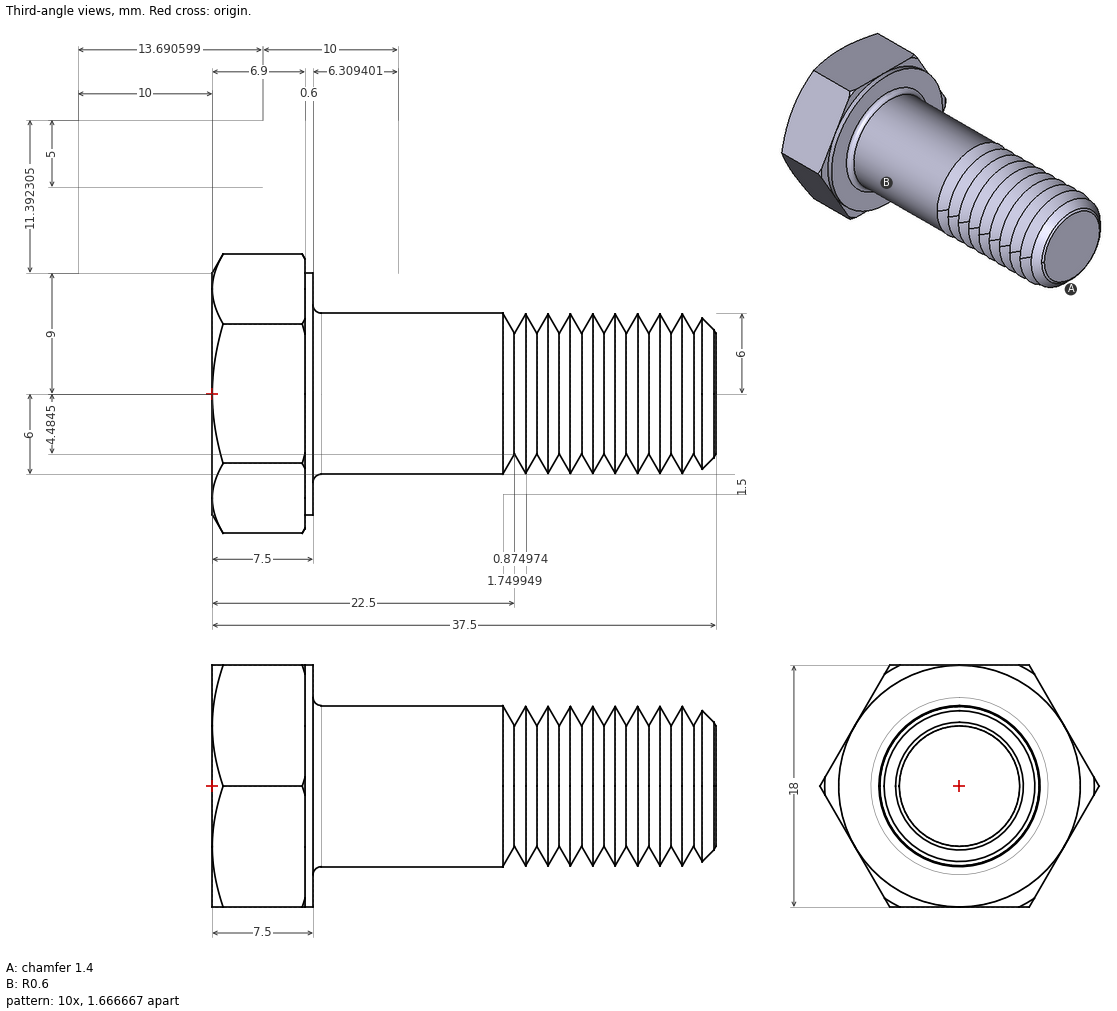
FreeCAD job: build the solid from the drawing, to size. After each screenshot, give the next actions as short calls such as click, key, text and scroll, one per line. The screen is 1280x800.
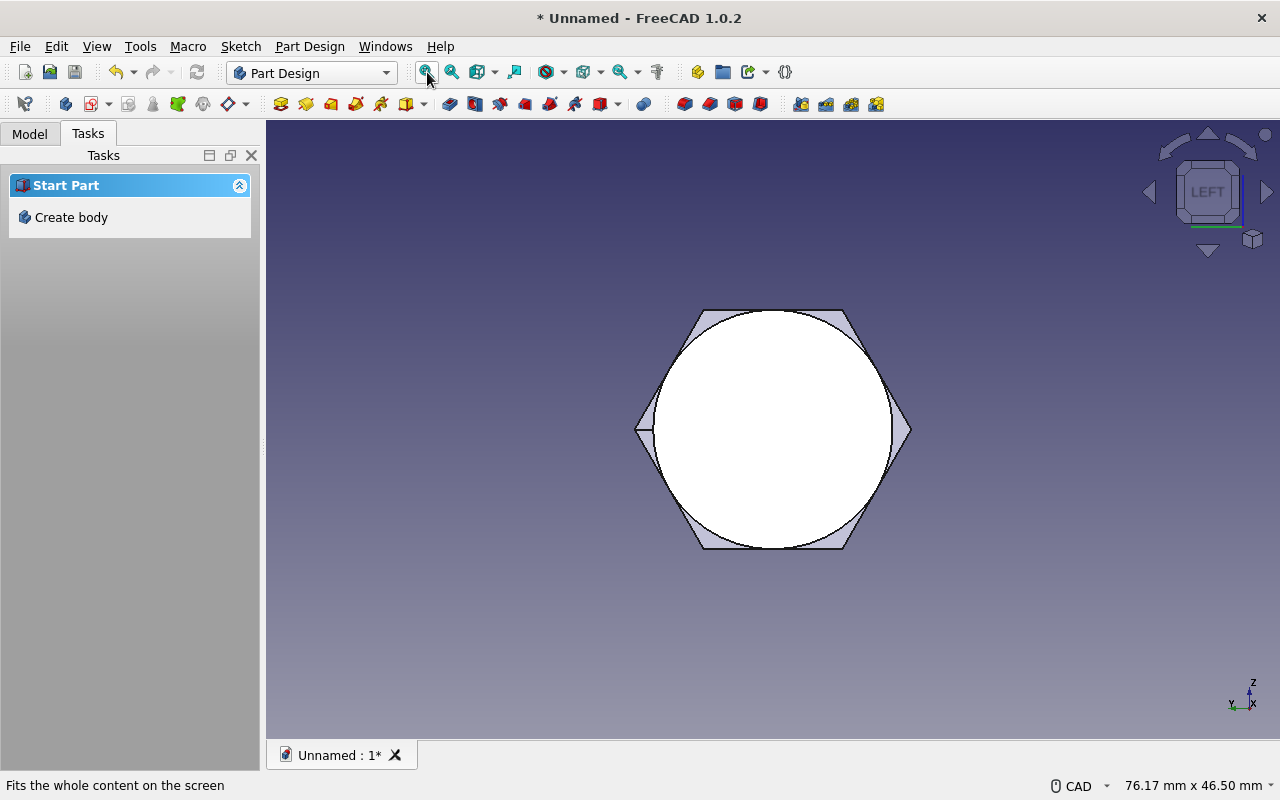
click(427, 72)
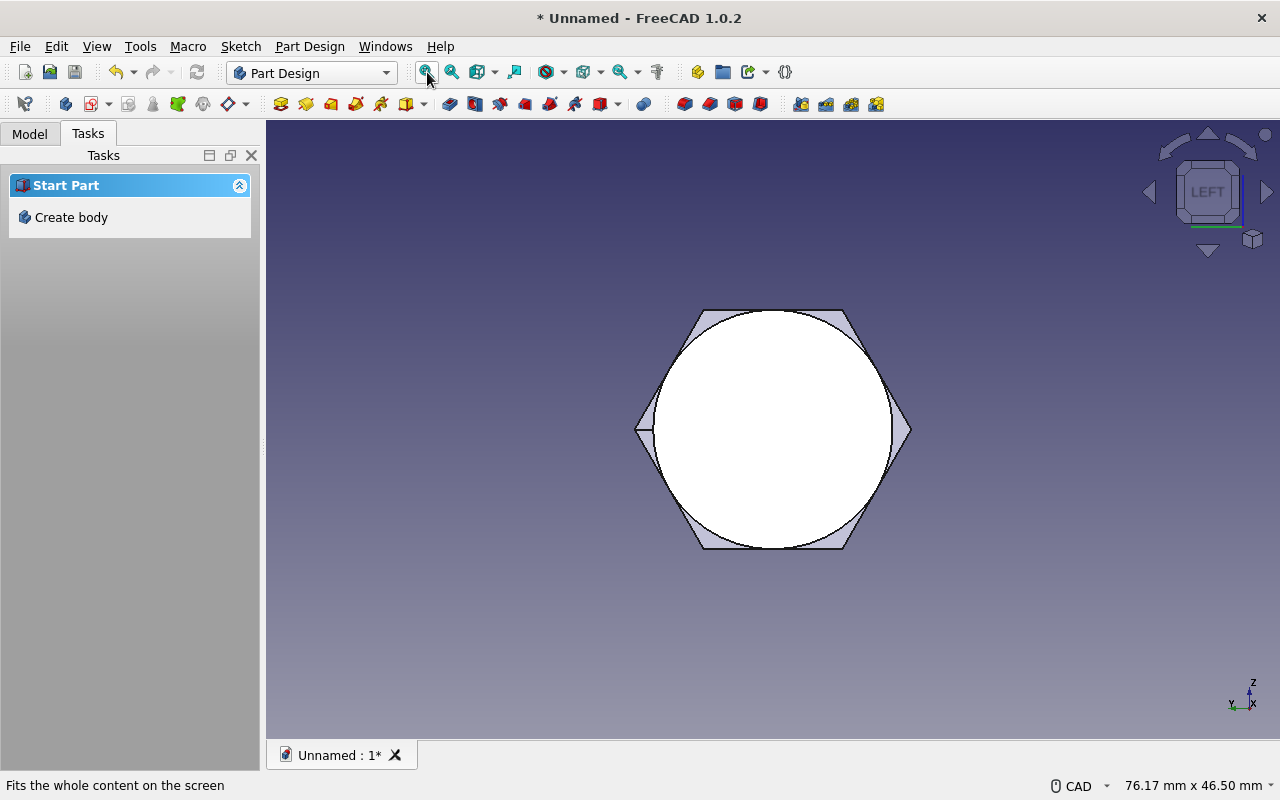
key(v)
key(3)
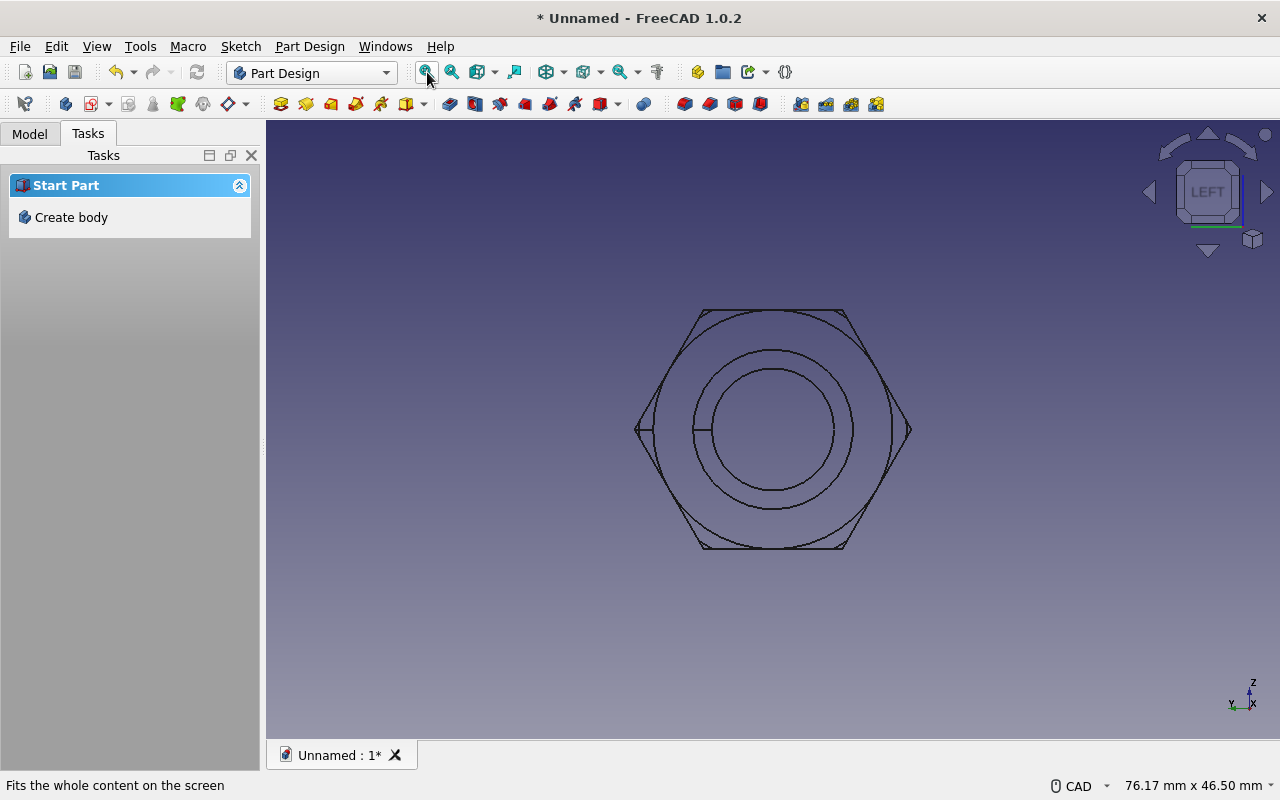
key(0)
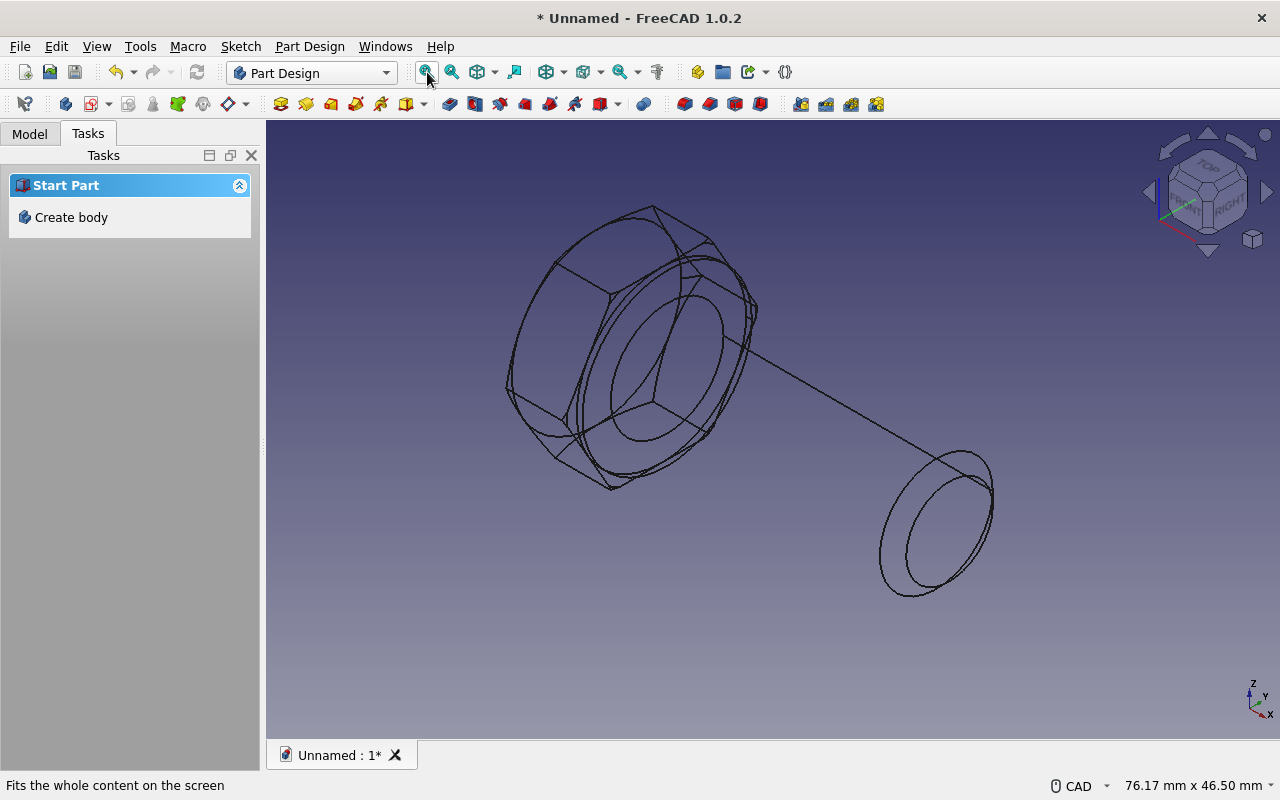
click(611, 400)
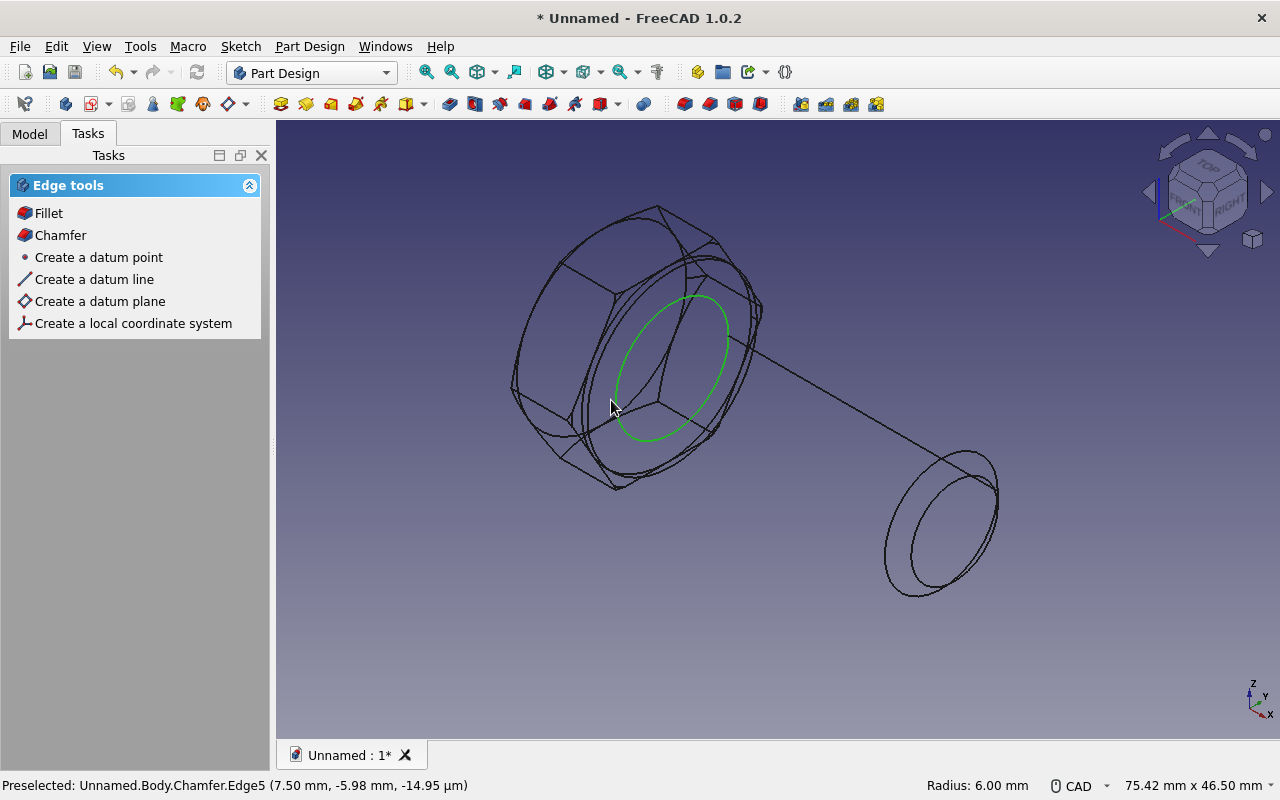
key(v)
key(1)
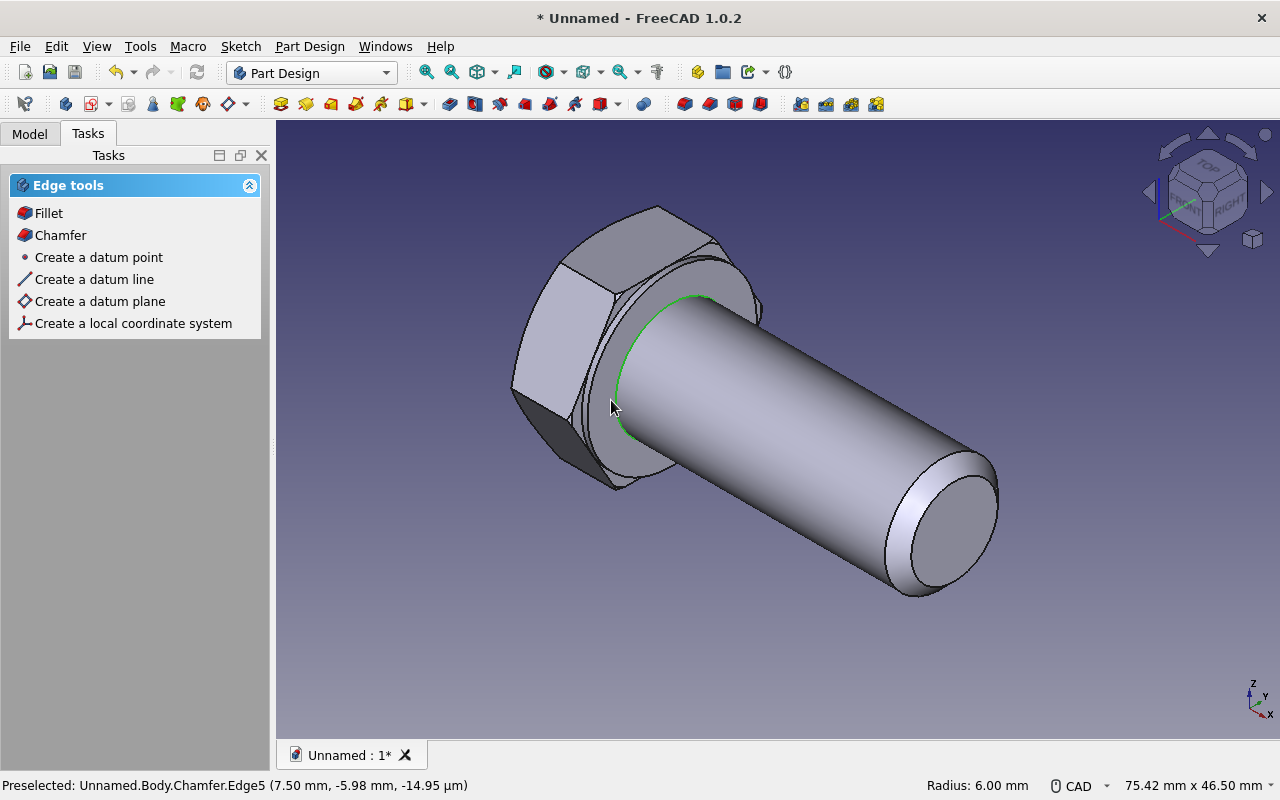
click(685, 104)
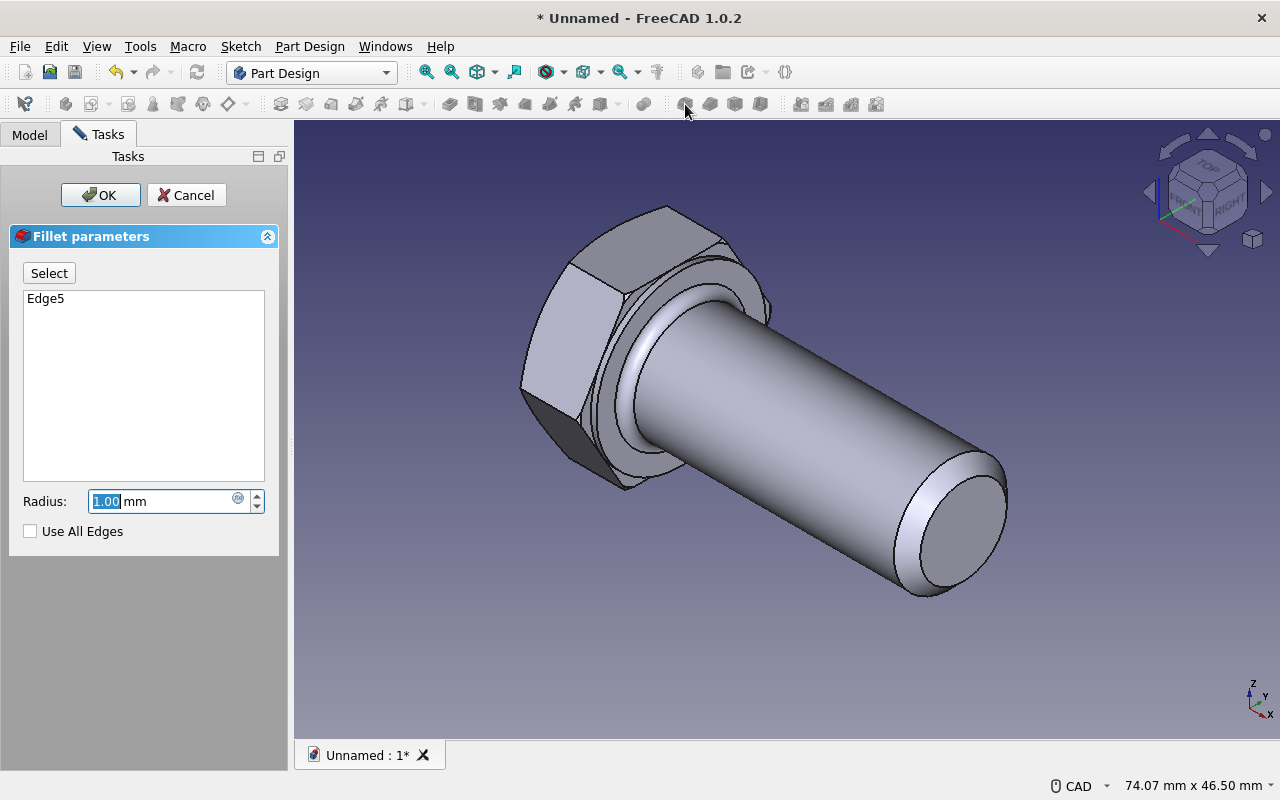
text(0.6)
key(Tab)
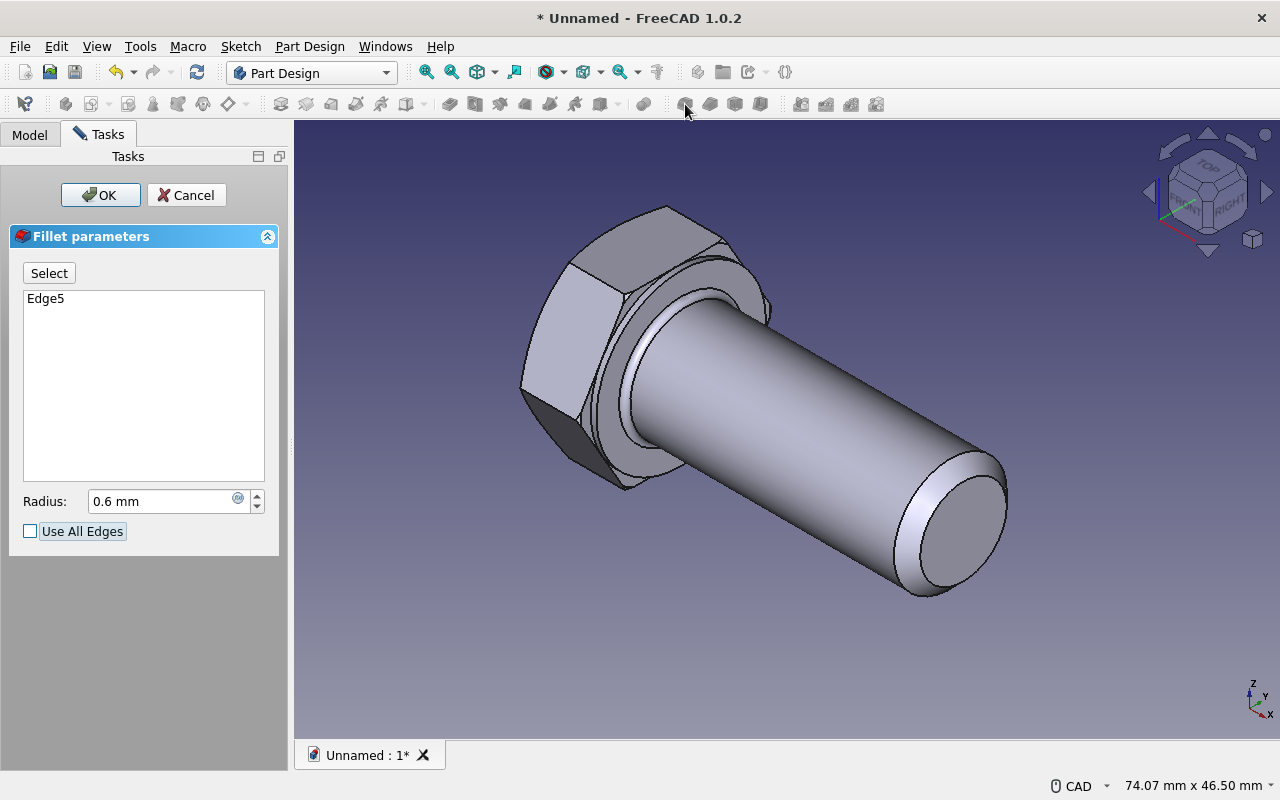
click(101, 195)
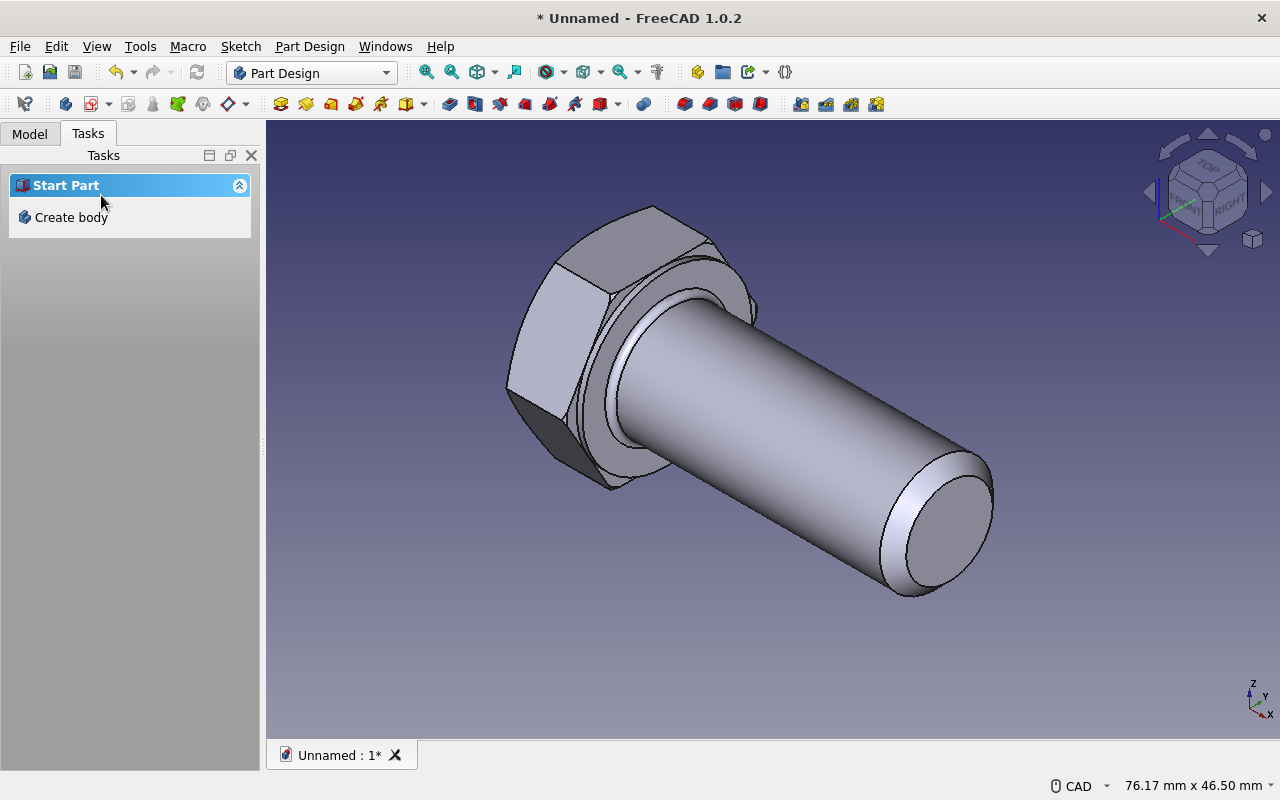
click(90, 104)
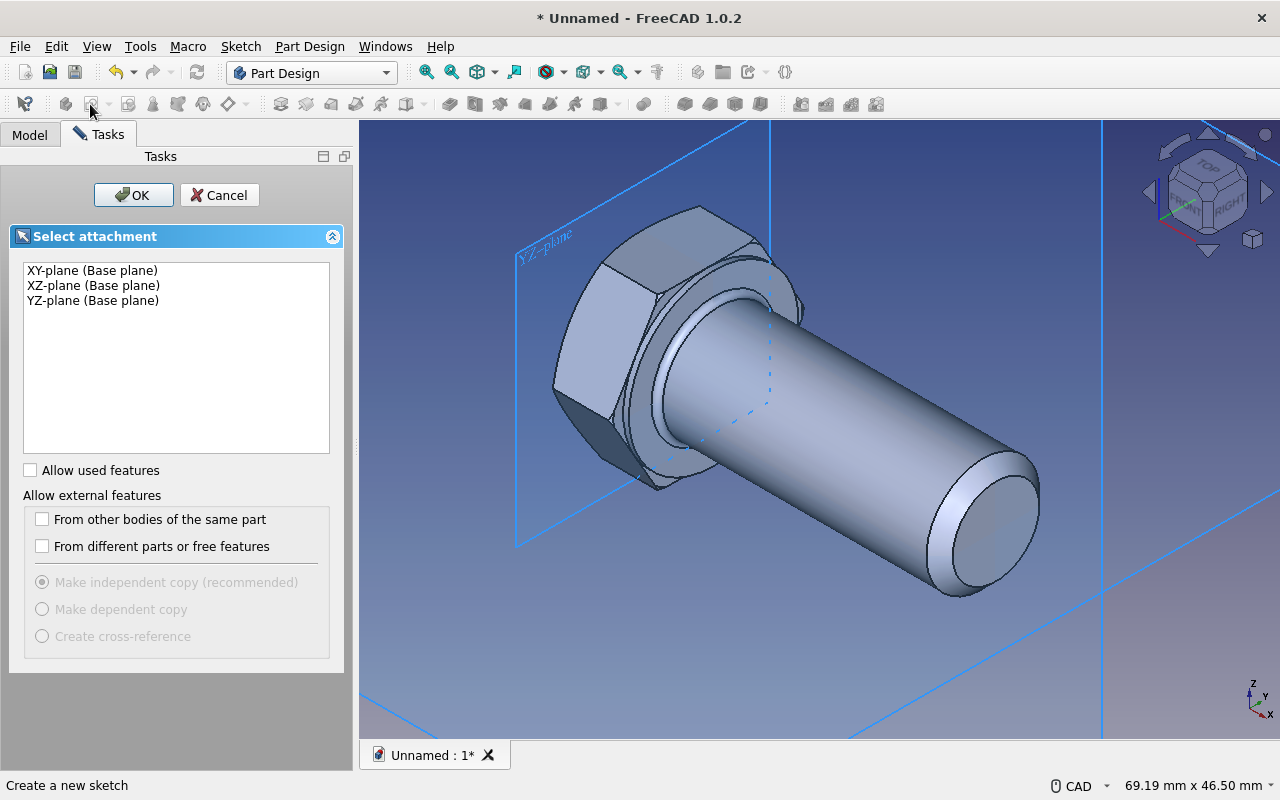
click(84, 270)